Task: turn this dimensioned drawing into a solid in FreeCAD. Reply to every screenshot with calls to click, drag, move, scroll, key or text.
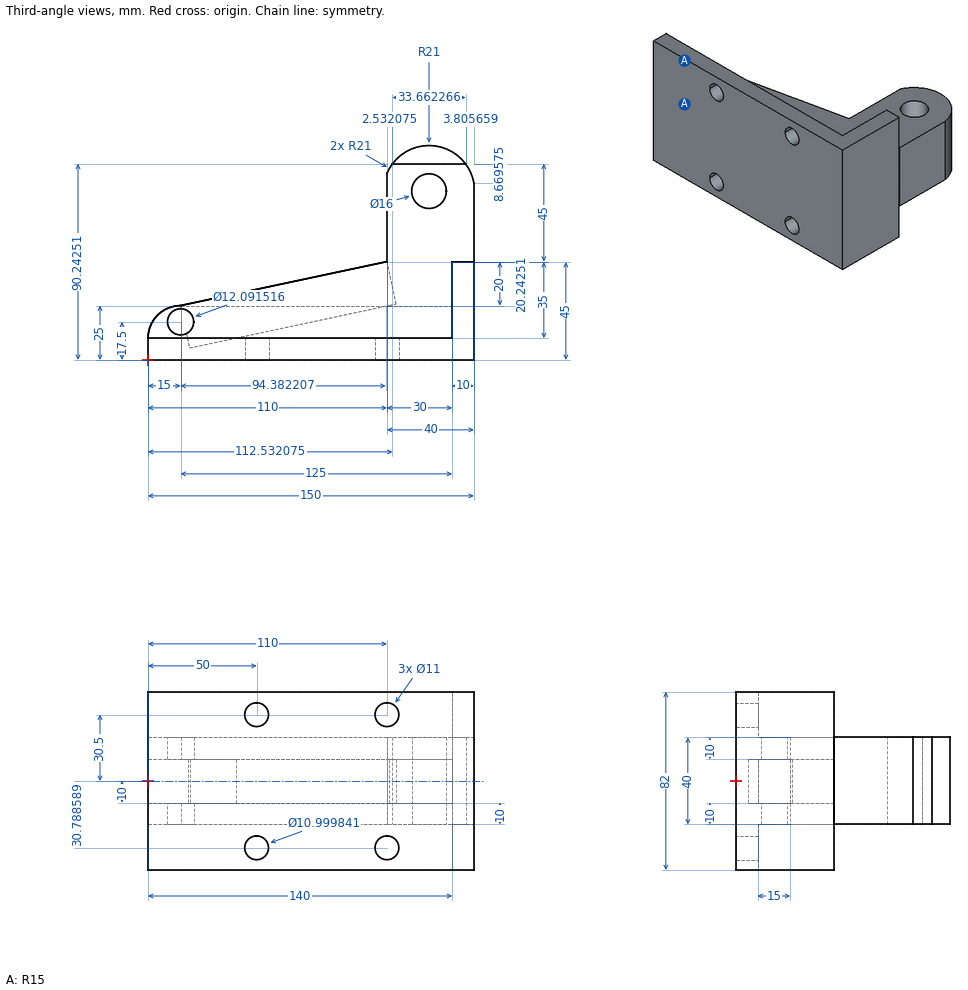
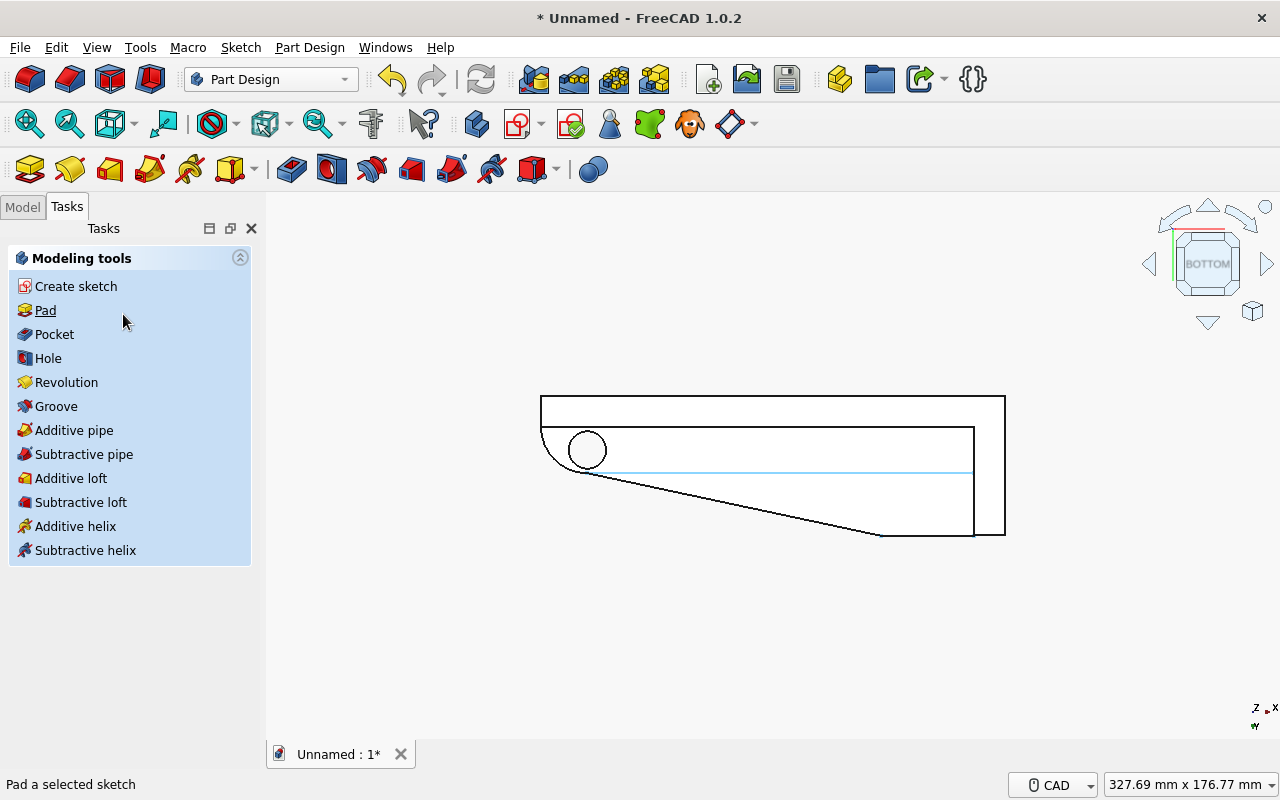
click(30, 170)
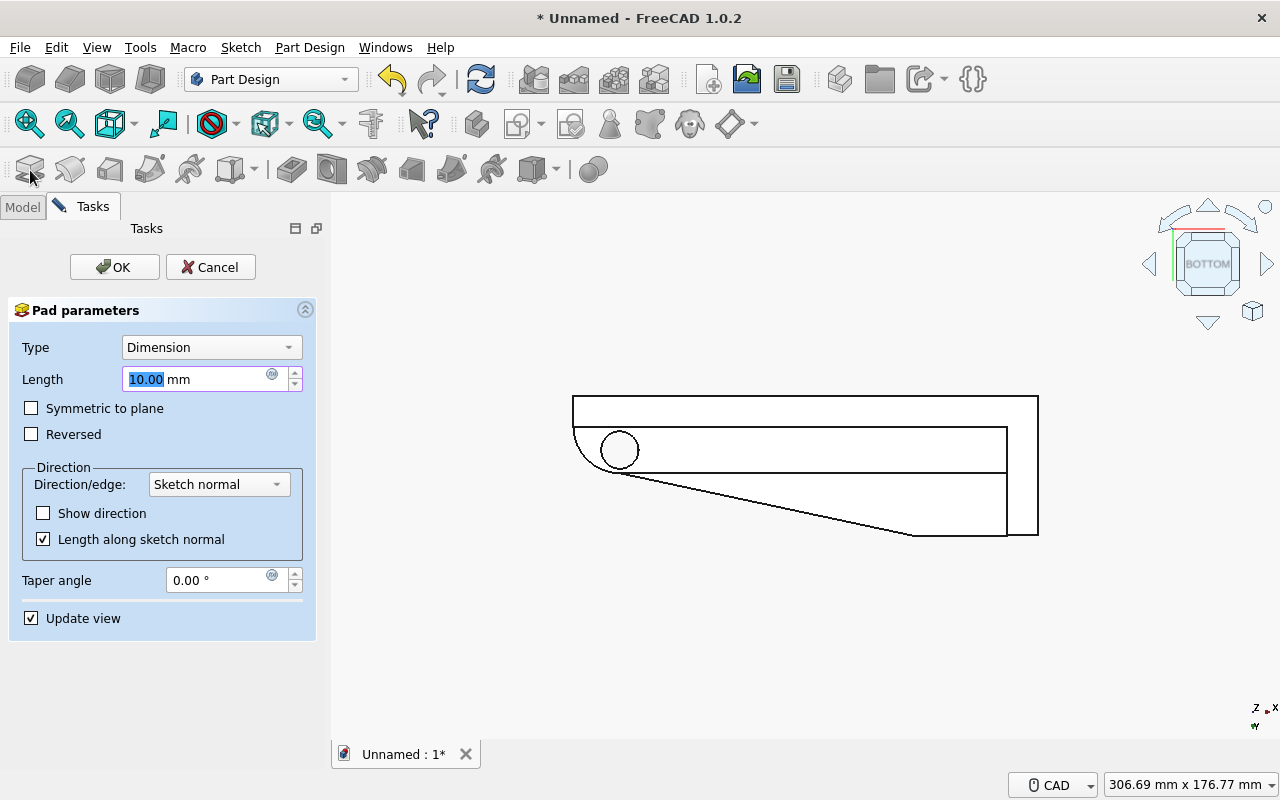
text(40)
key(Tab)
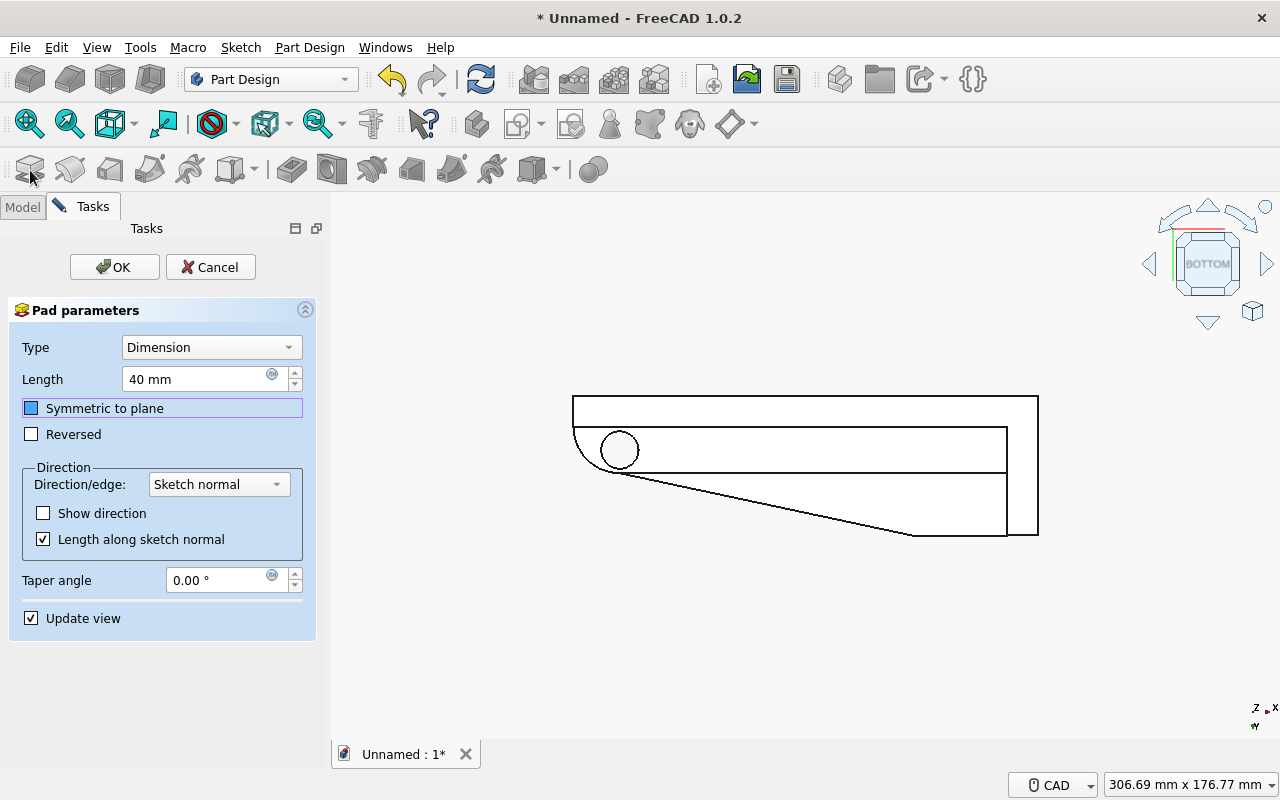
click(30, 434)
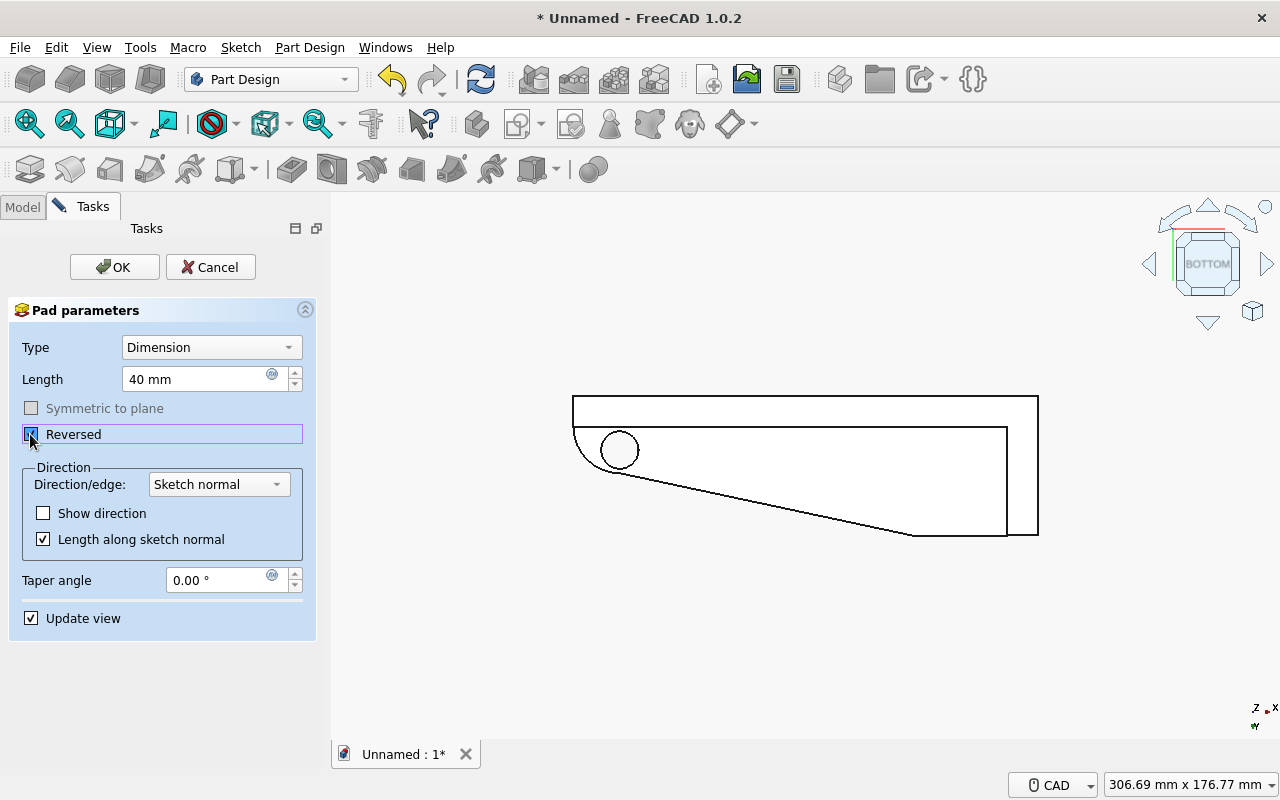
click(115, 267)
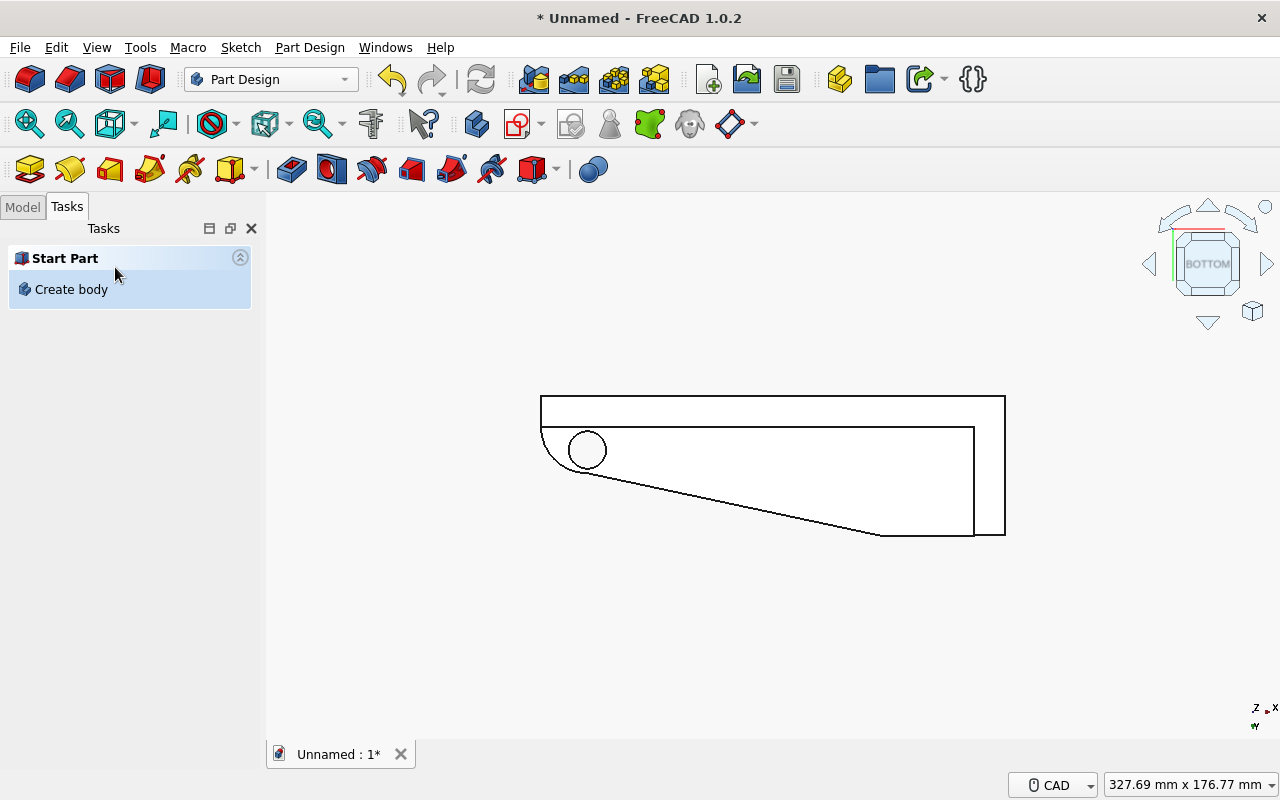
key(0)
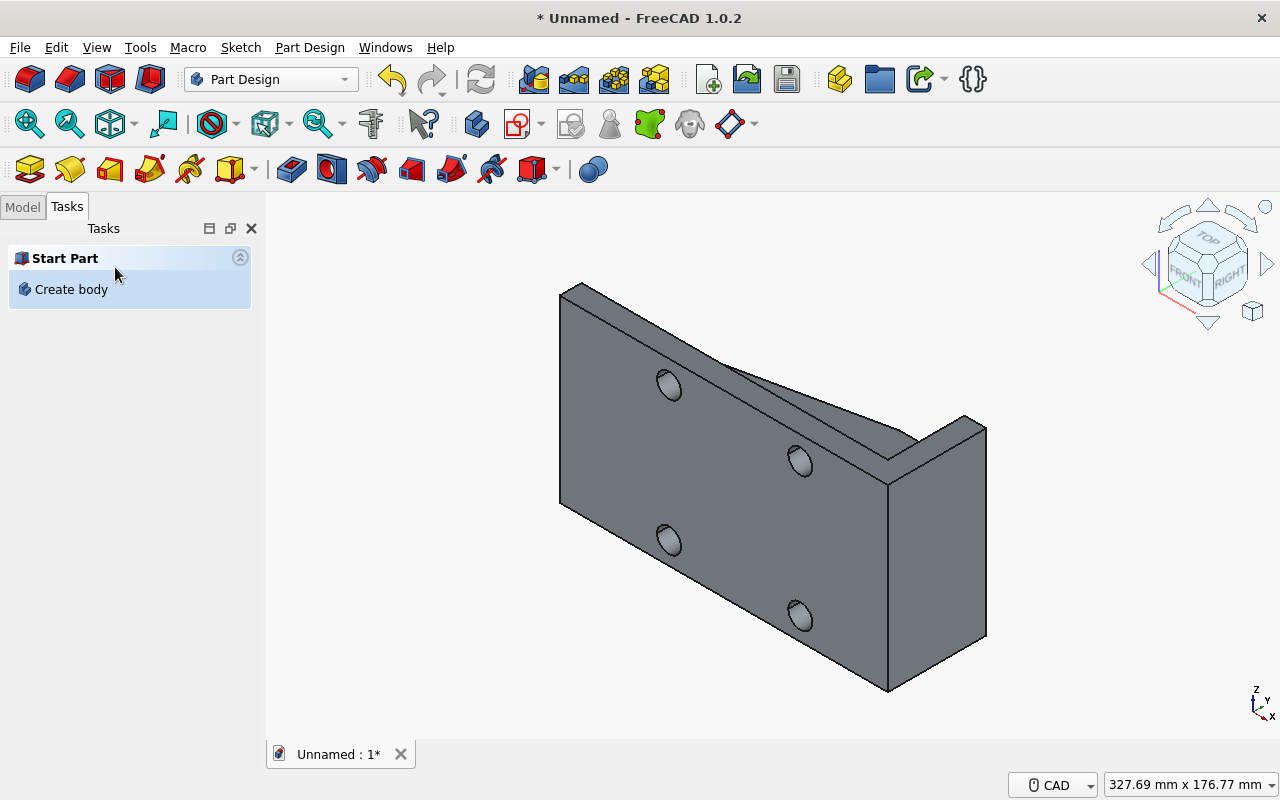
key(2)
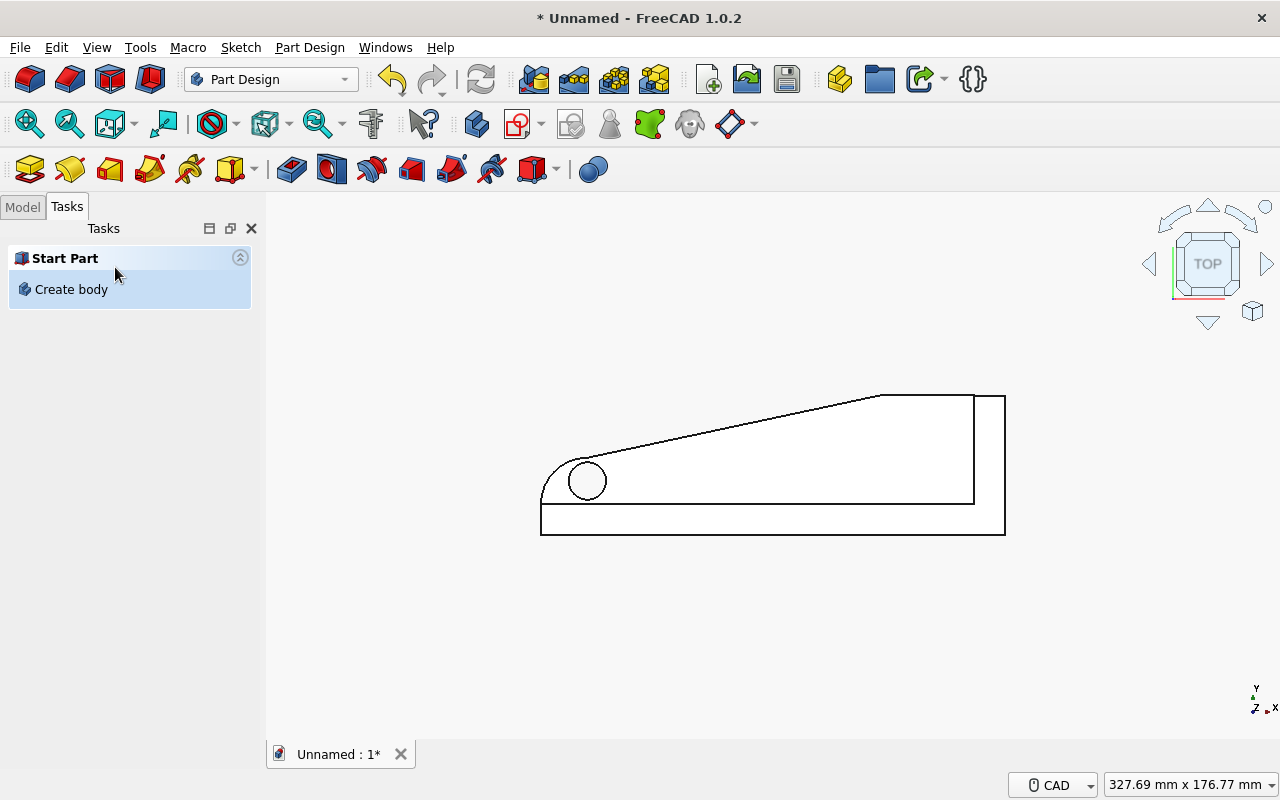
click(881, 449)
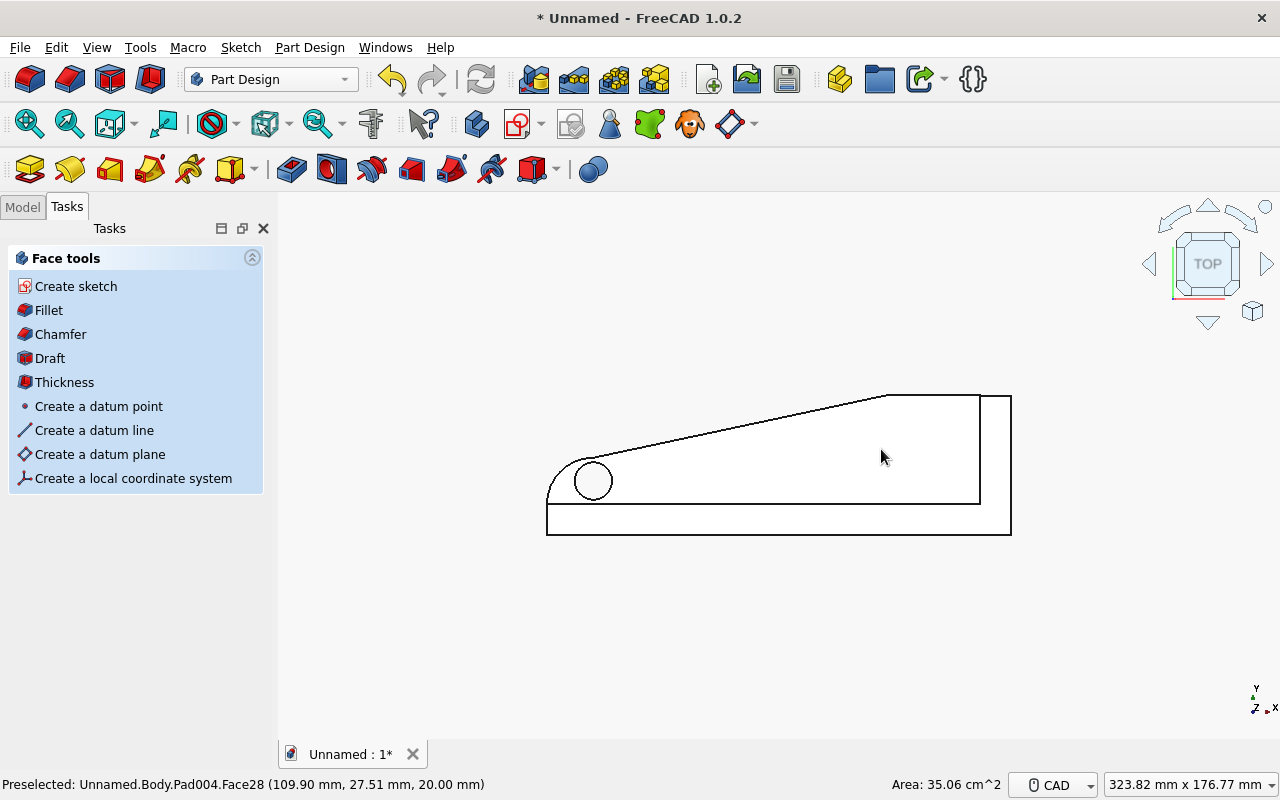
click(518, 124)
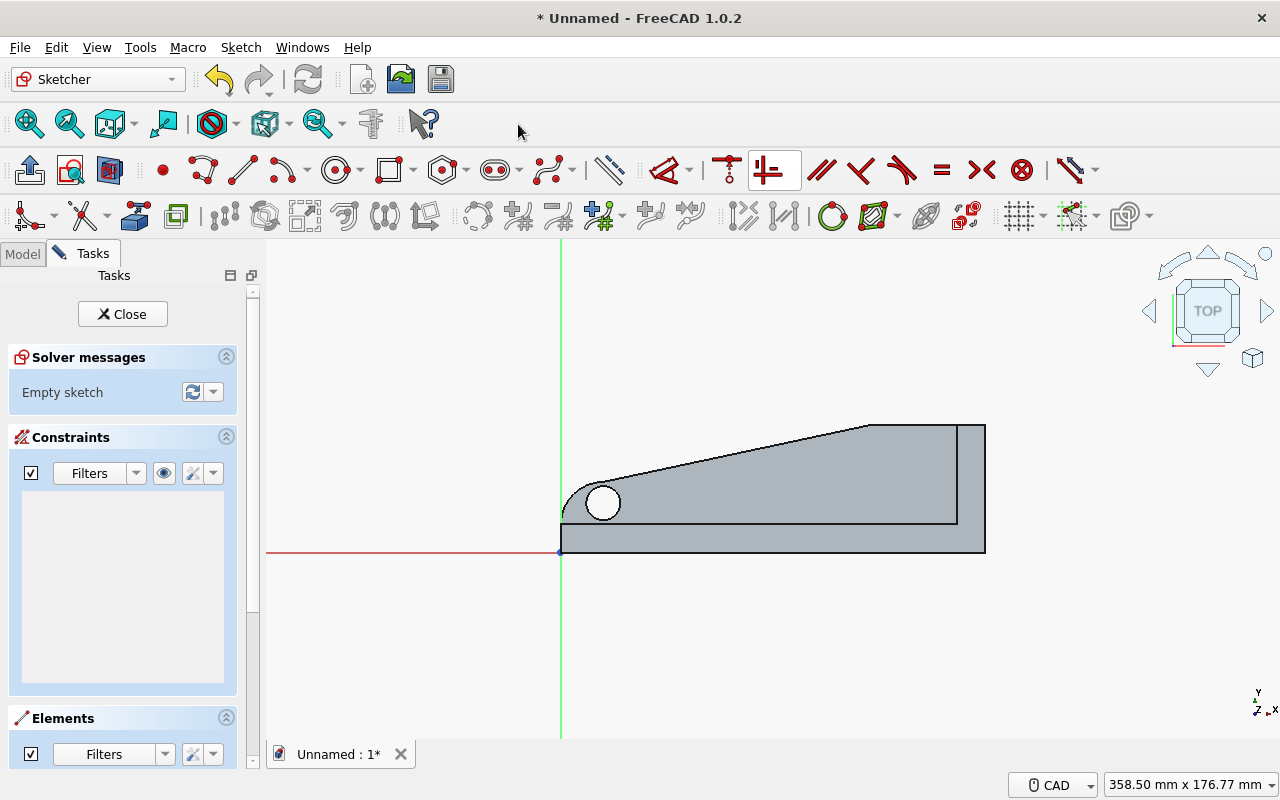
scroll(1059, 287, up, 5)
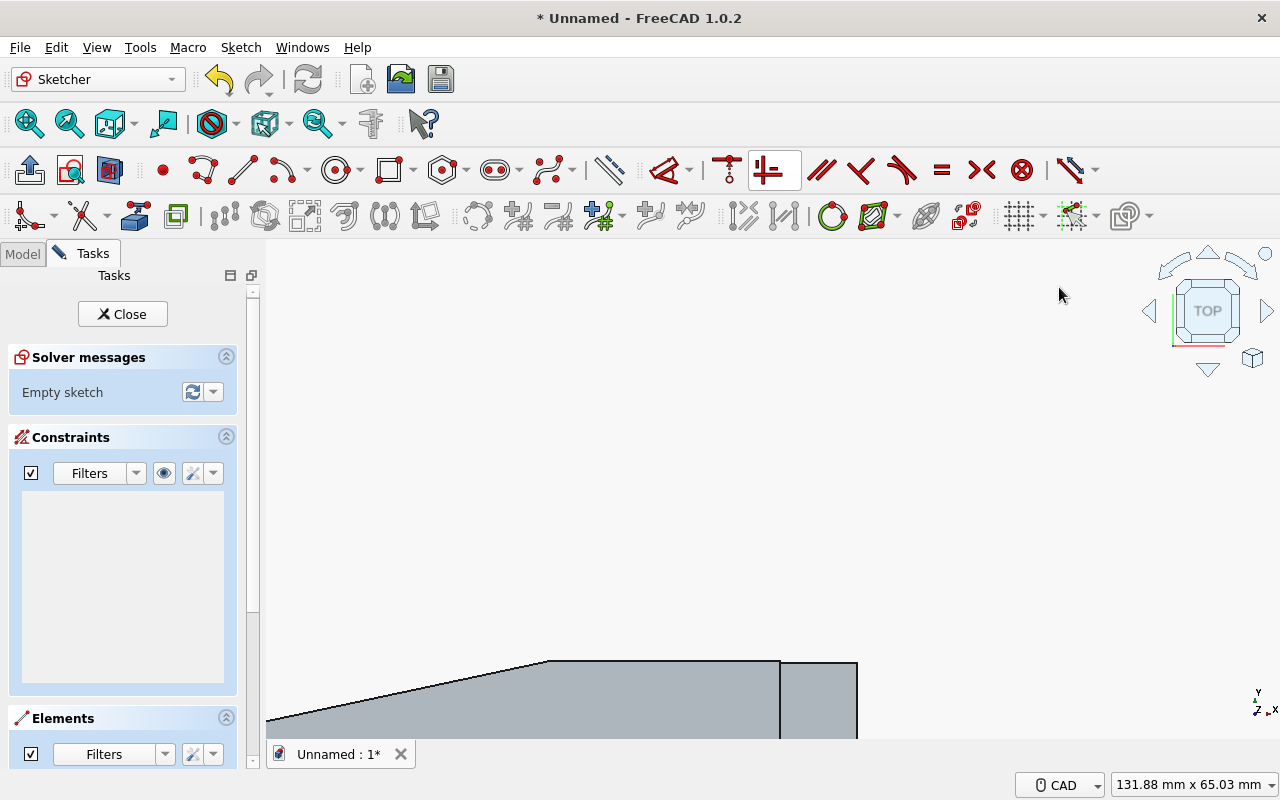
key(g)
key(r)